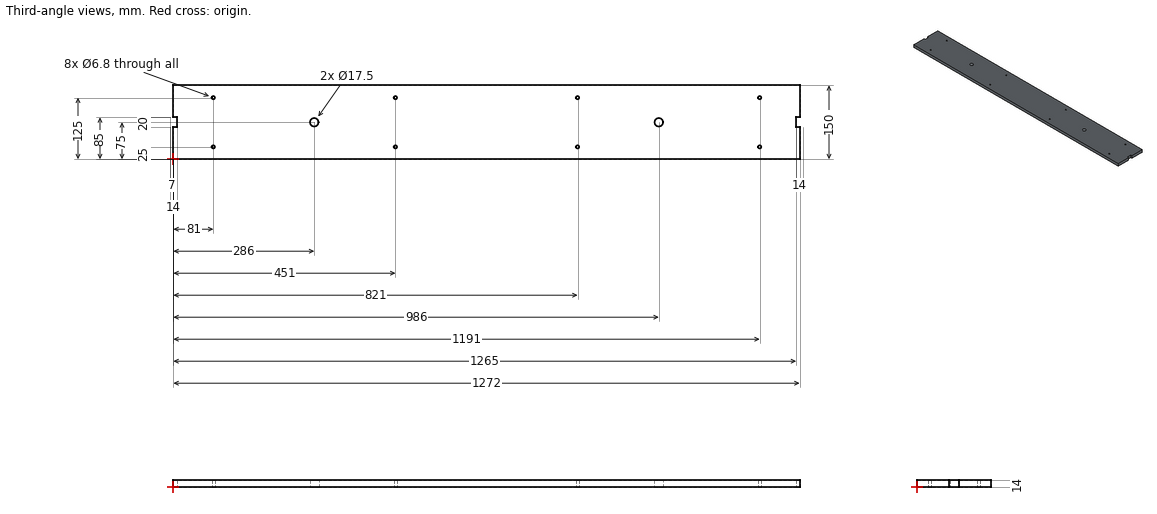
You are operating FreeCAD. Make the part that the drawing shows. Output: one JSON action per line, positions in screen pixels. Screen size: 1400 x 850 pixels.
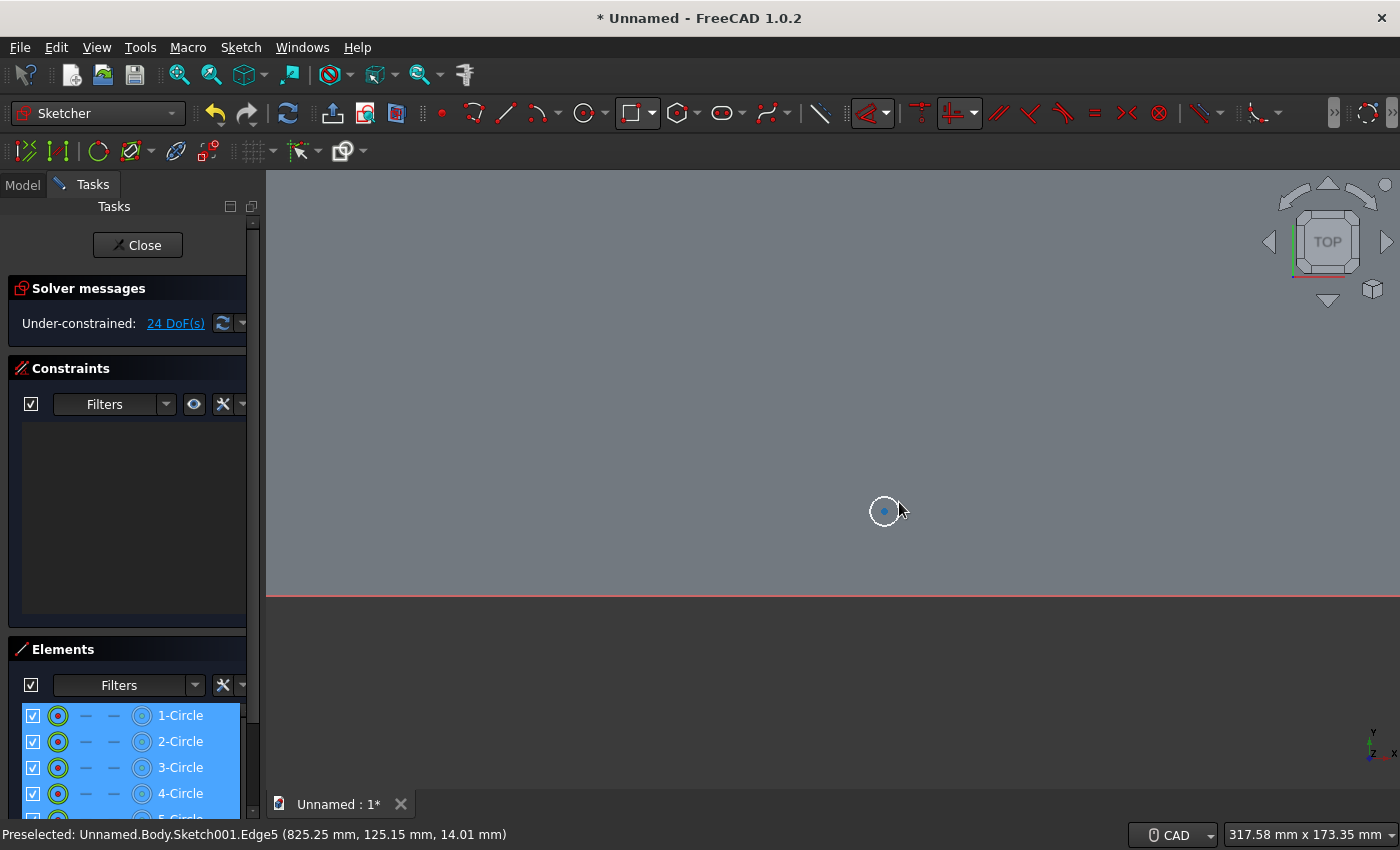
{"action": "left_click", "coordinate": [895, 501]}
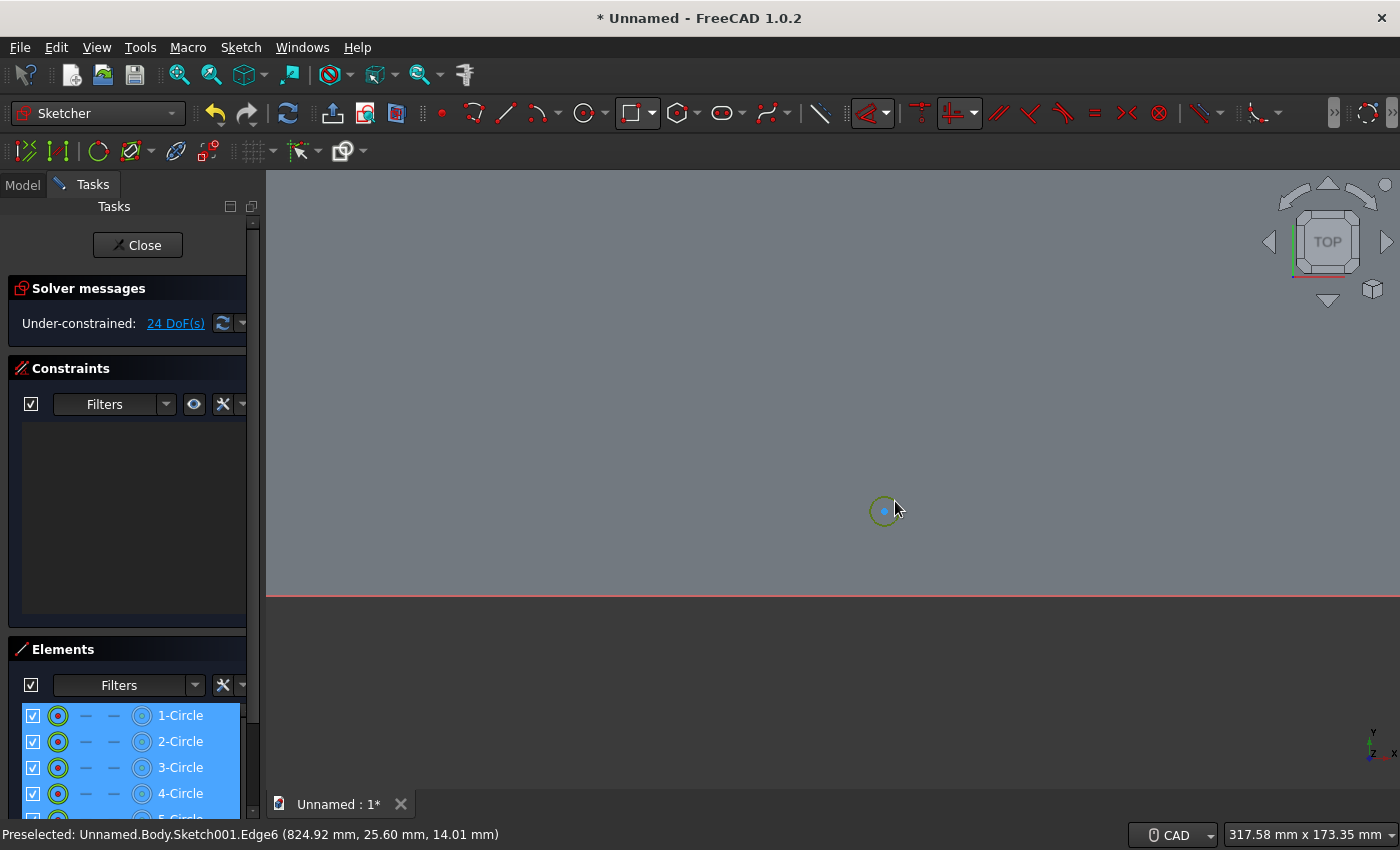
{"action": "scroll", "coordinate": [899, 502], "scroll_direction": "down", "scroll_amount": 9}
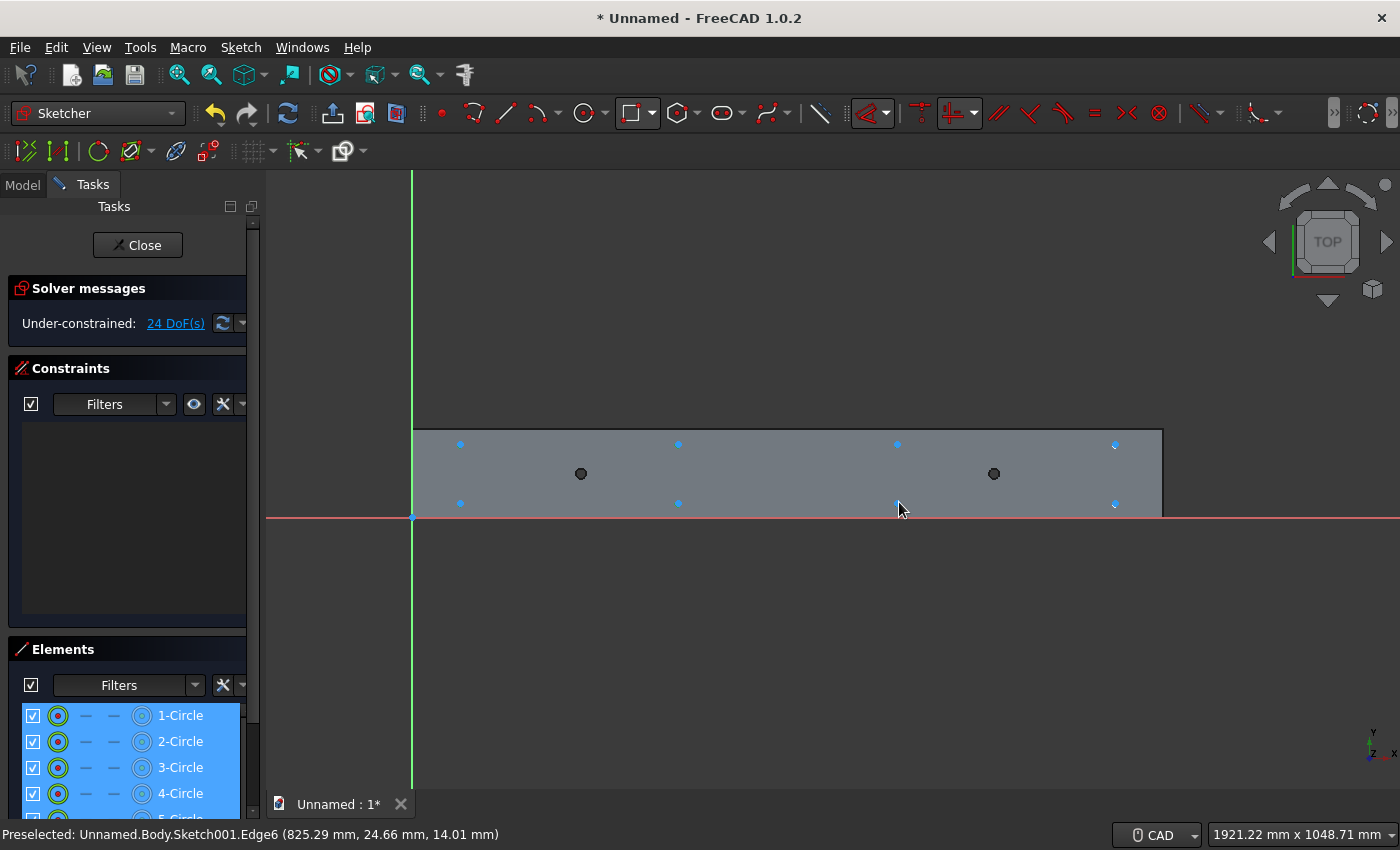
{"action": "scroll", "coordinate": [1117, 443], "scroll_direction": "up", "scroll_amount": 9}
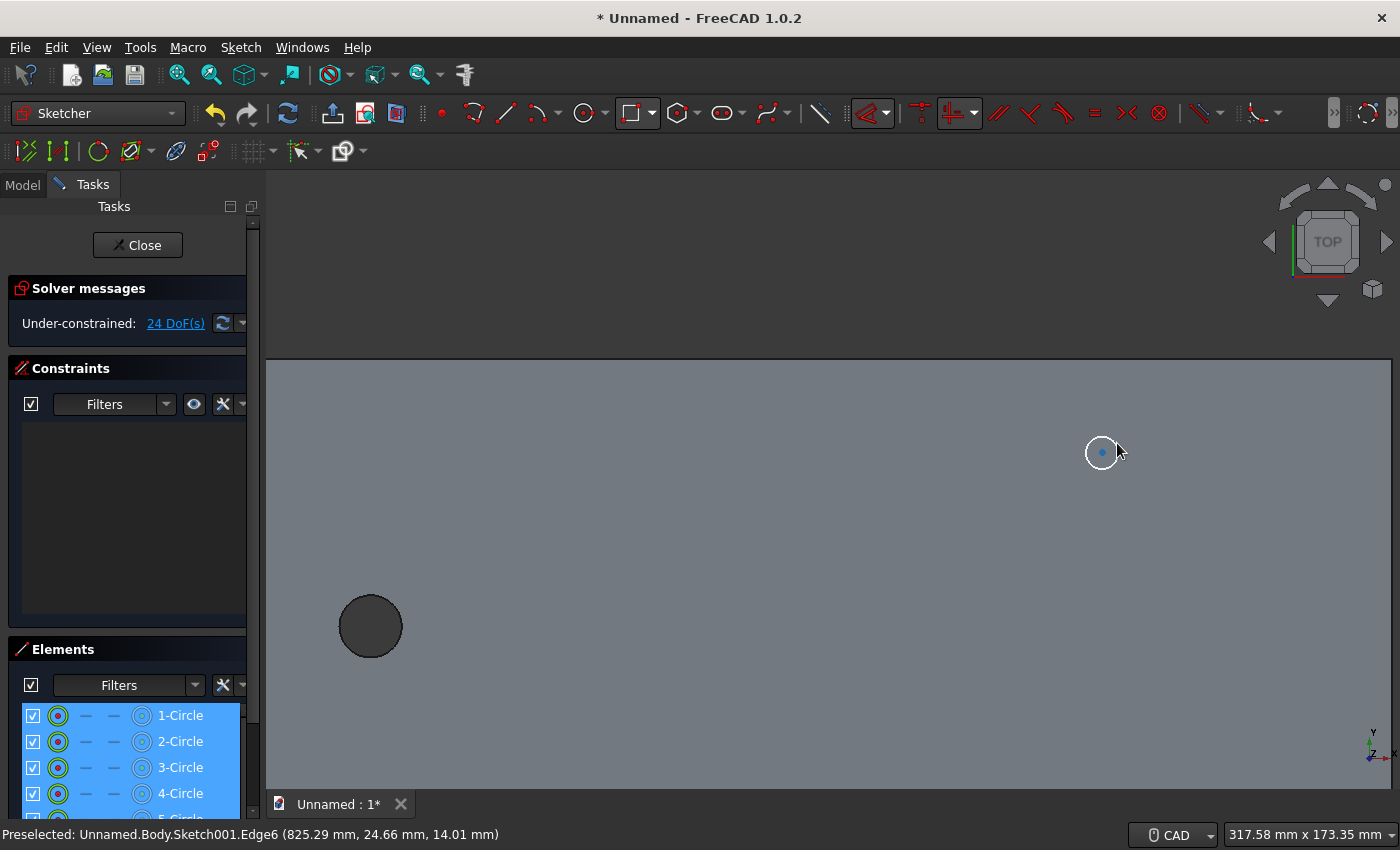
{"action": "left_click", "coordinate": [1113, 441]}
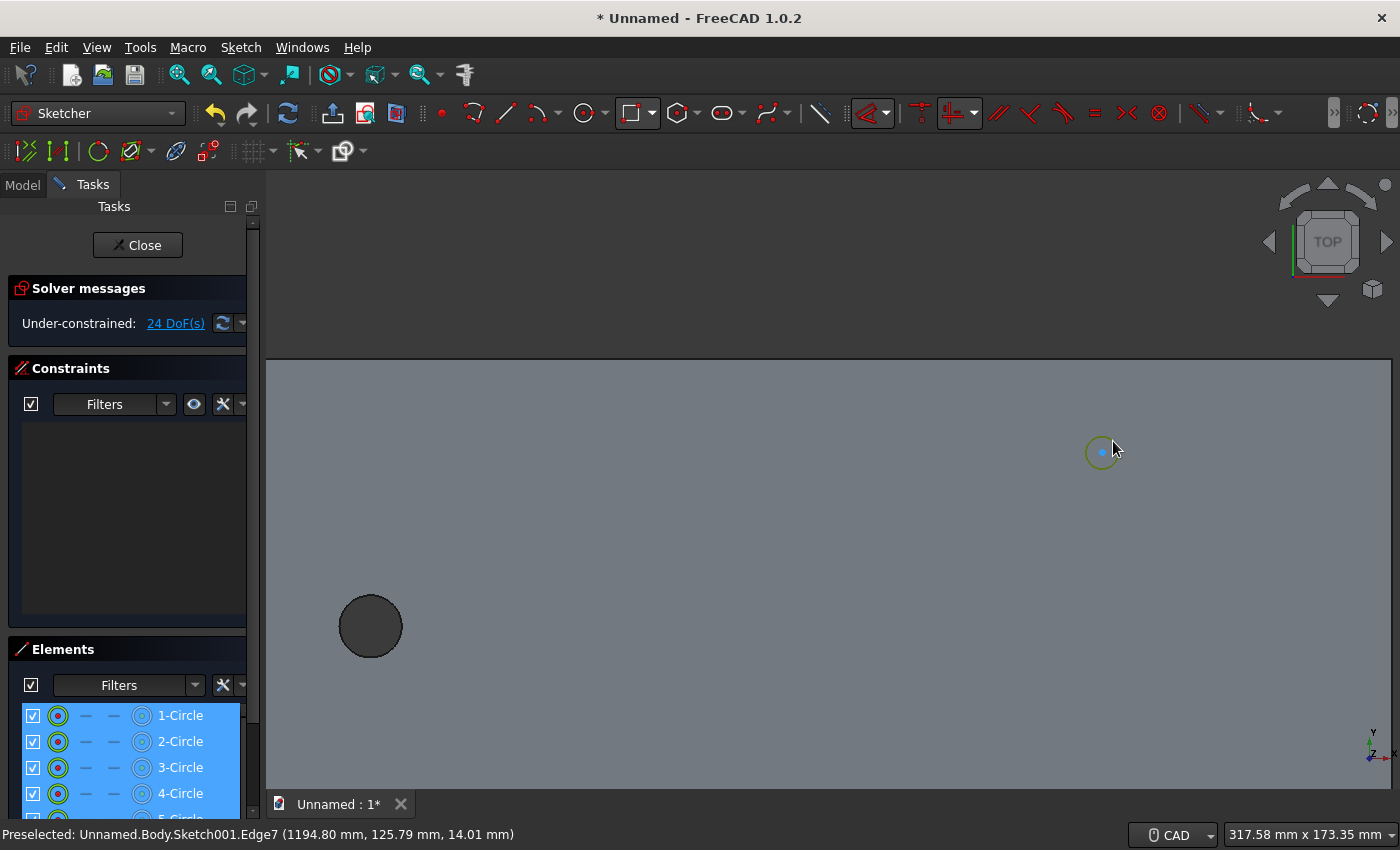
{"action": "scroll", "coordinate": [1117, 443], "scroll_direction": "down", "scroll_amount": 9}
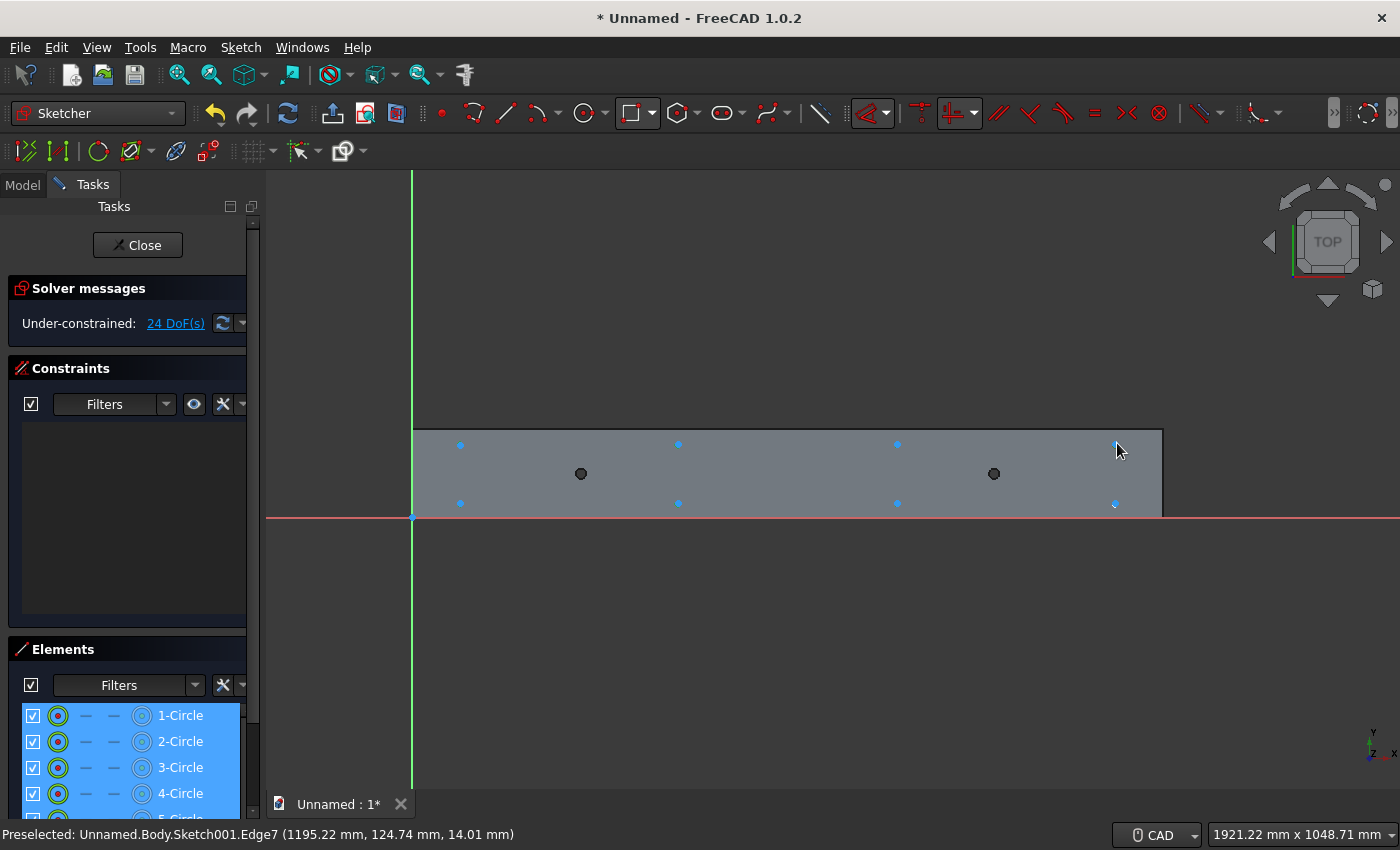
{"action": "scroll", "coordinate": [1117, 502], "scroll_direction": "up", "scroll_amount": 9}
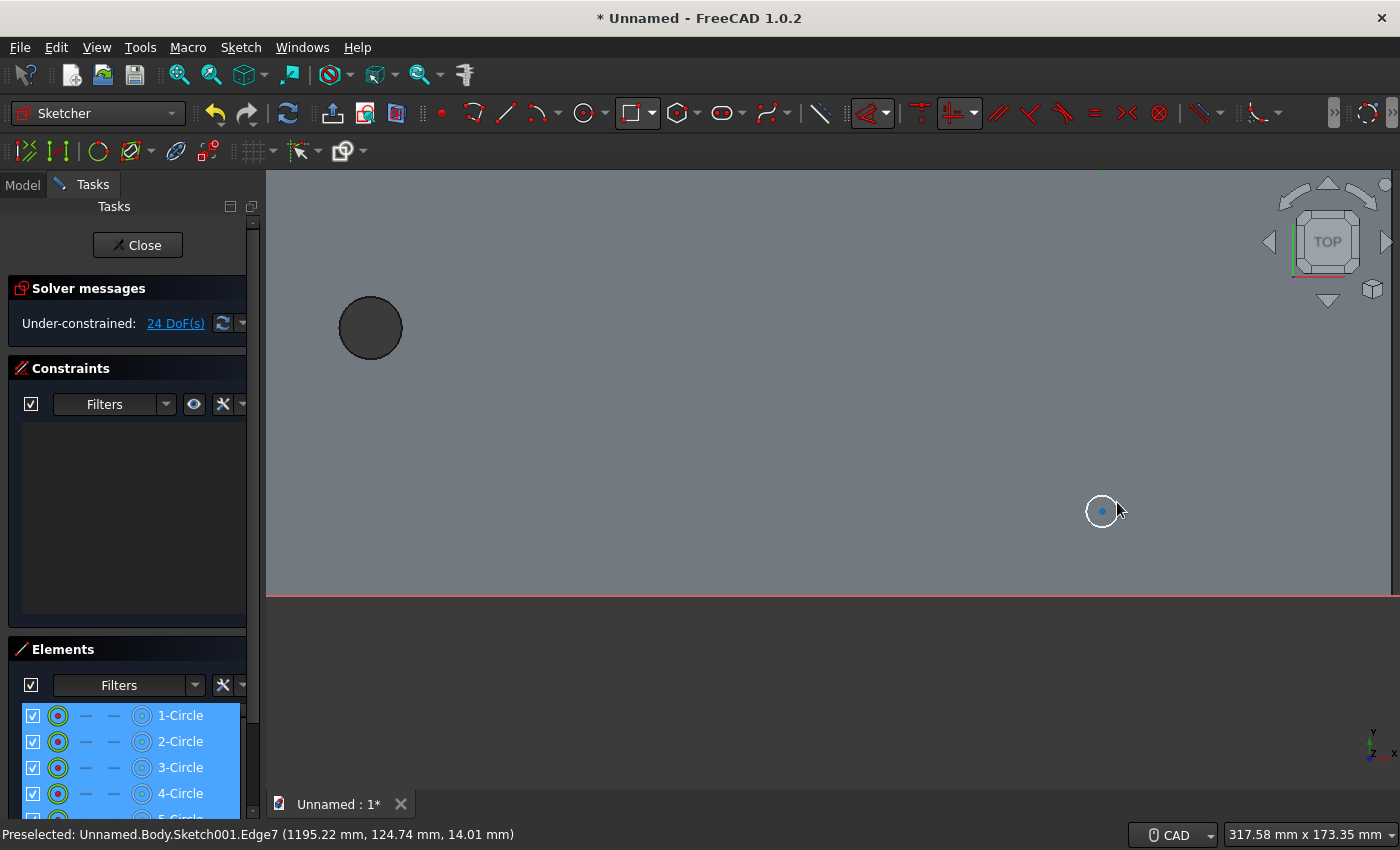
{"action": "left_click", "coordinate": [1113, 500]}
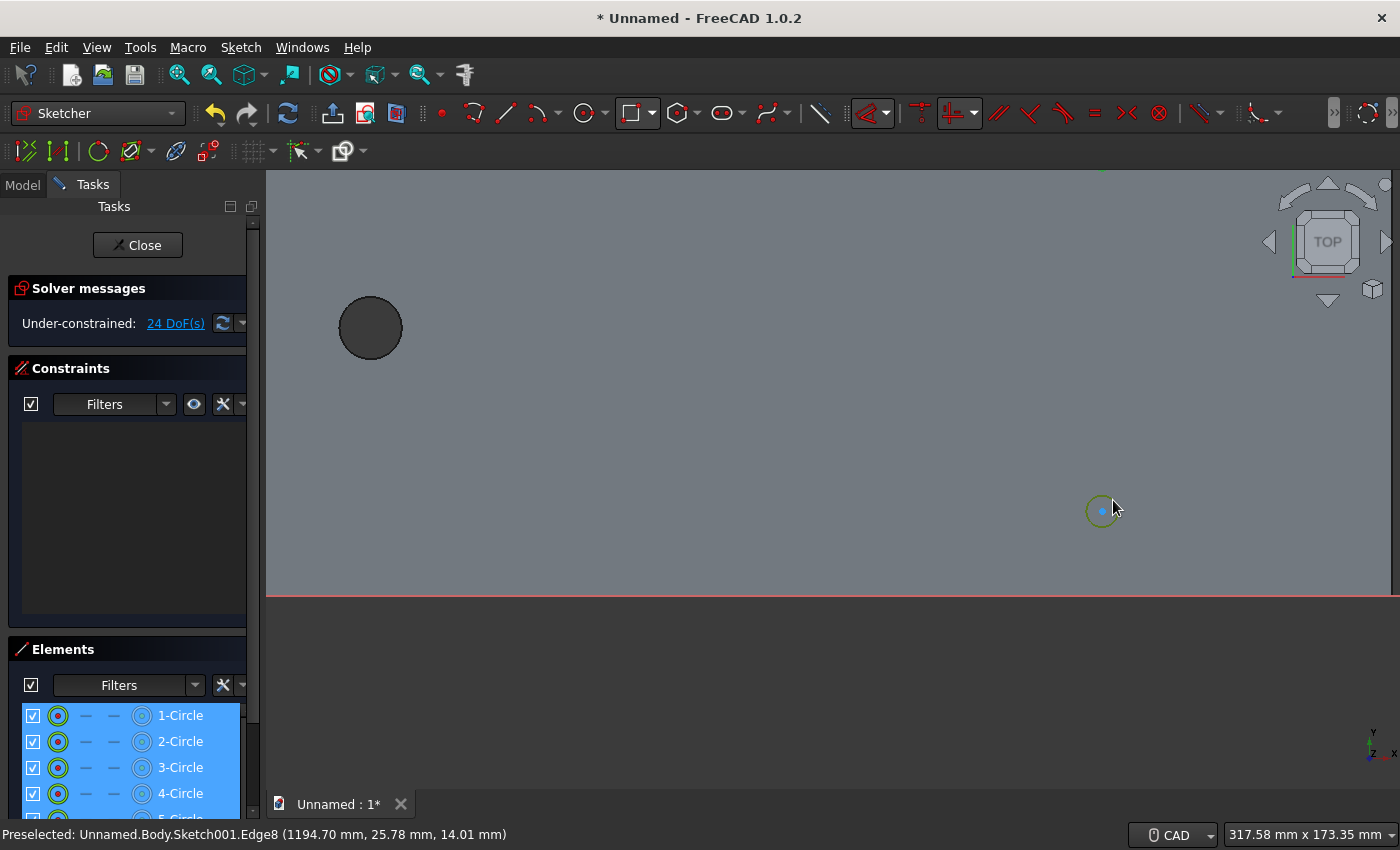
{"action": "left_click", "coordinate": [1096, 114]}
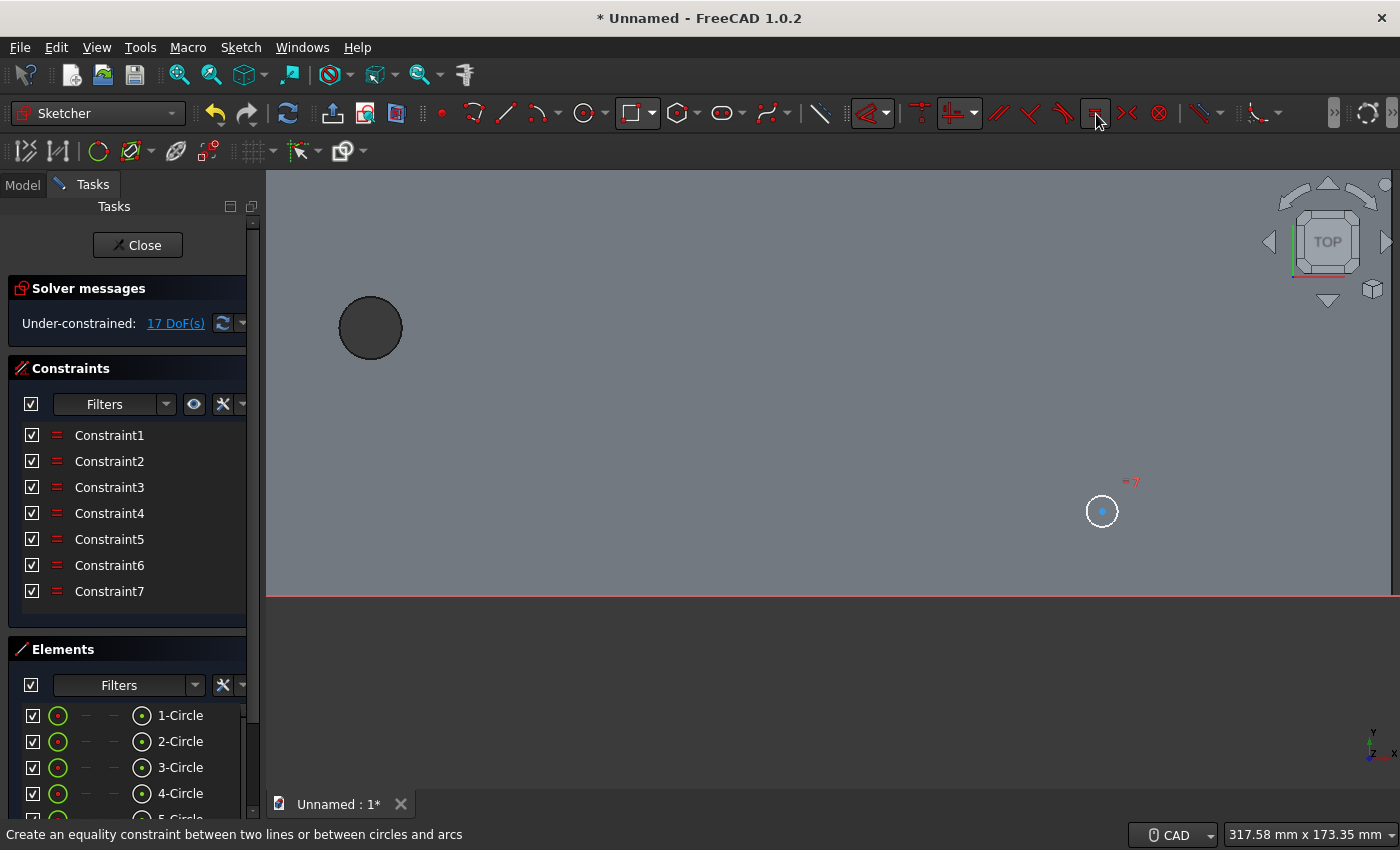
{"action": "scroll", "coordinate": [1117, 502], "scroll_direction": "down", "scroll_amount": 9}